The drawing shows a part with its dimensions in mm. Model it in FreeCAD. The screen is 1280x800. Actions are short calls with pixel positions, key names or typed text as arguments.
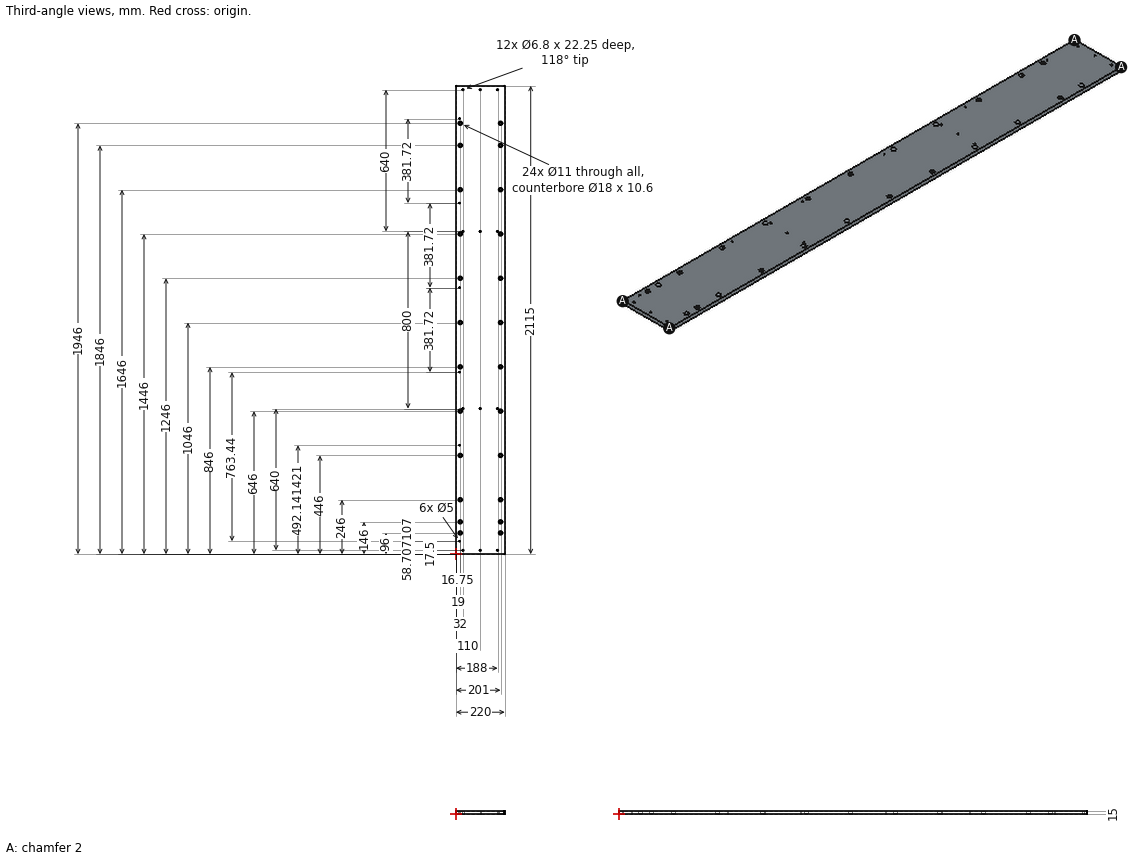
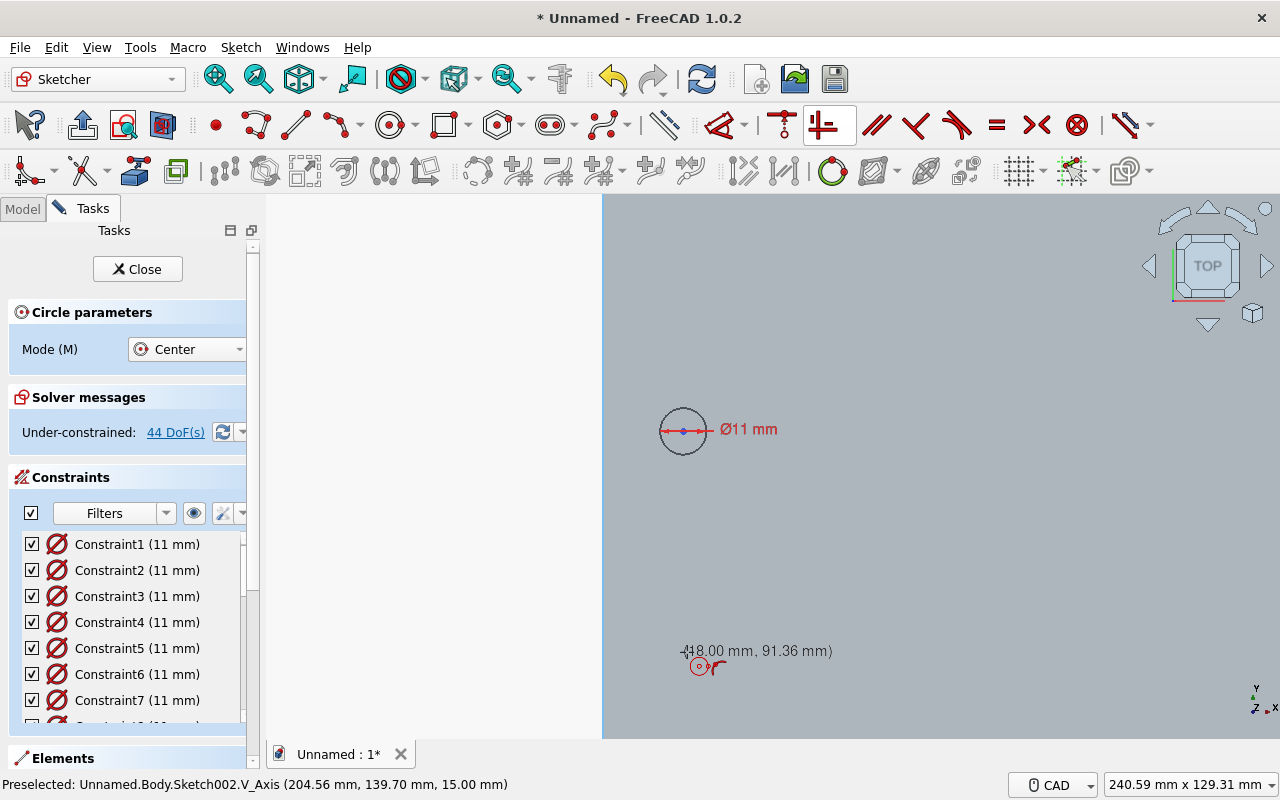
scroll(687, 652, down, 15)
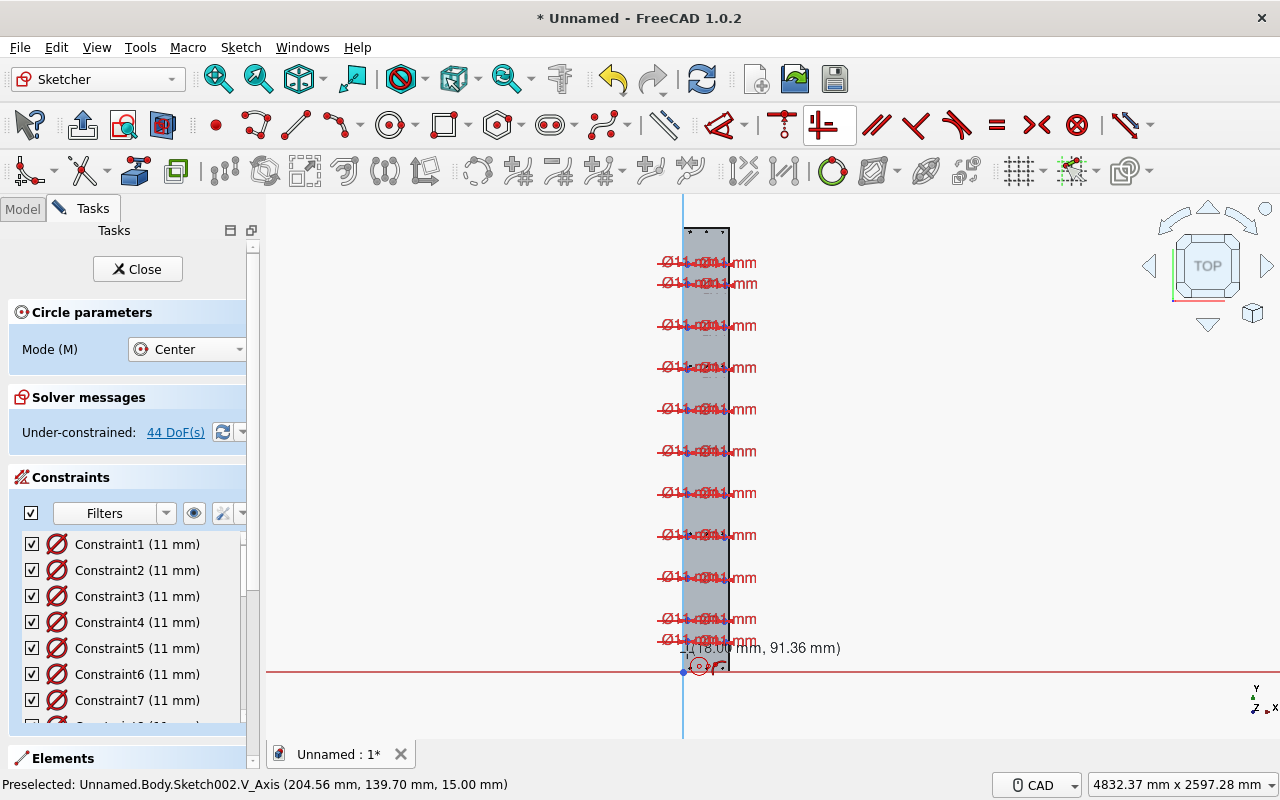
scroll(687, 652, up, 7)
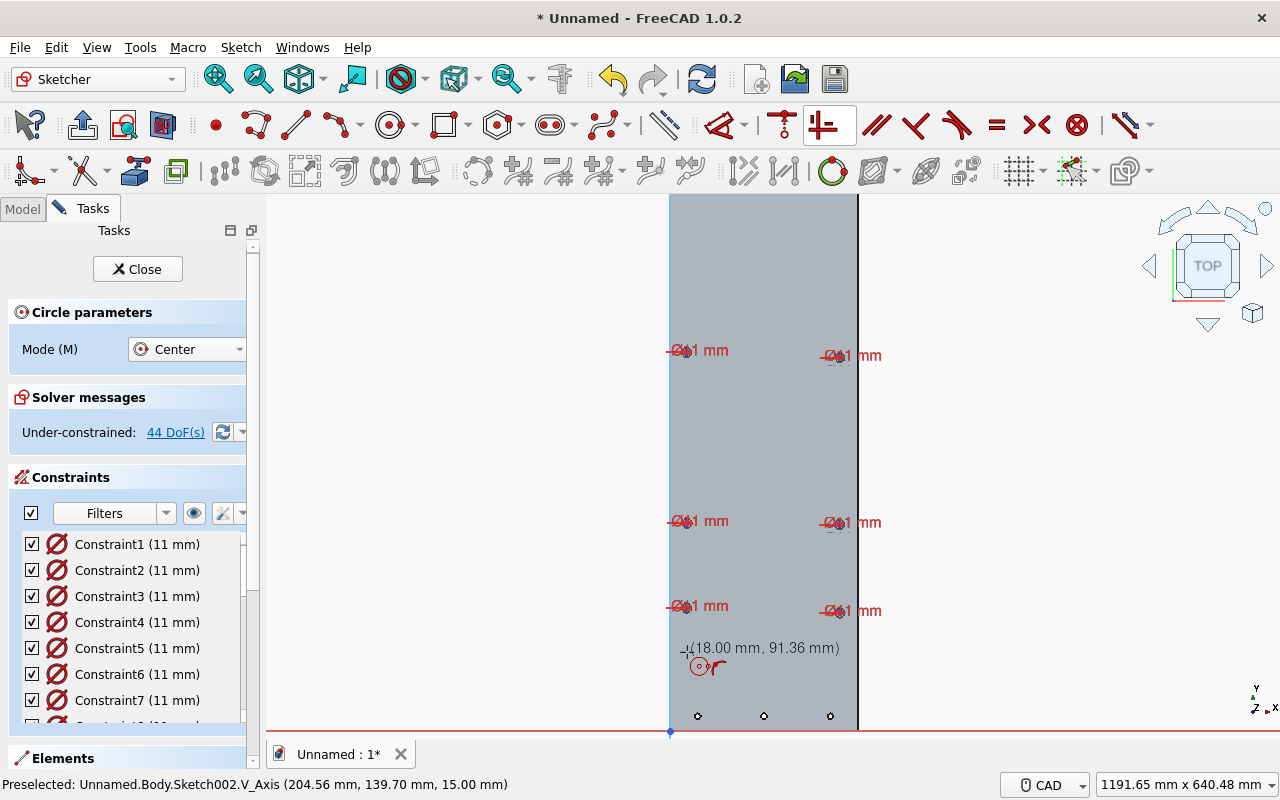
click(687, 650)
move(690, 646)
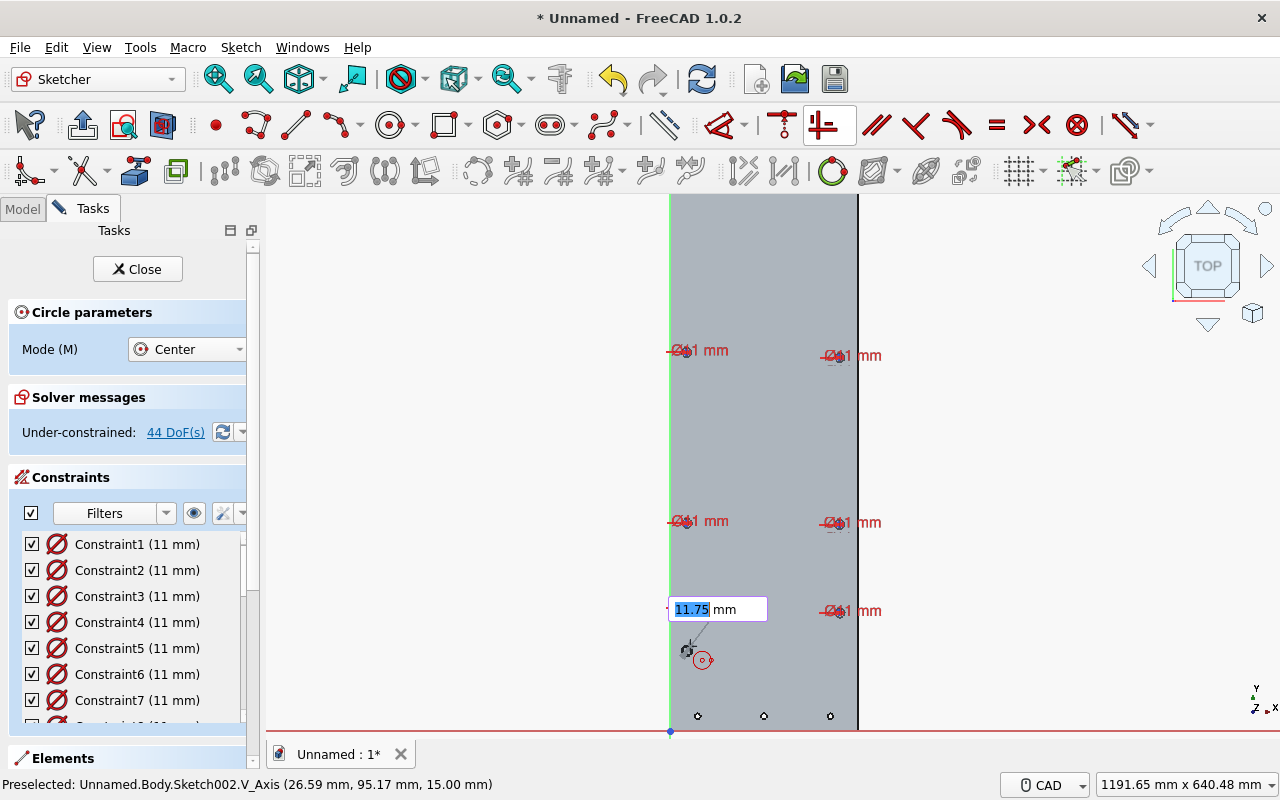
text(11)
key(Return)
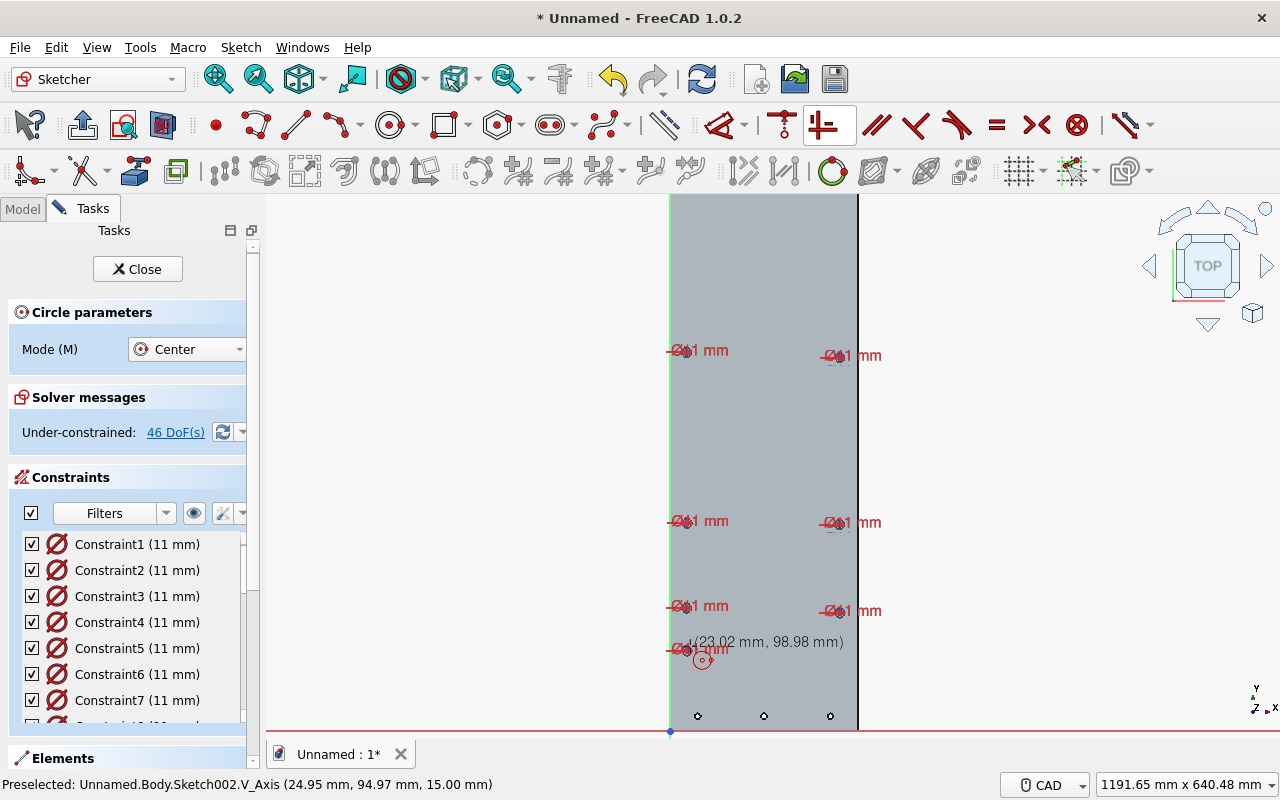
scroll(841, 650, up, 8)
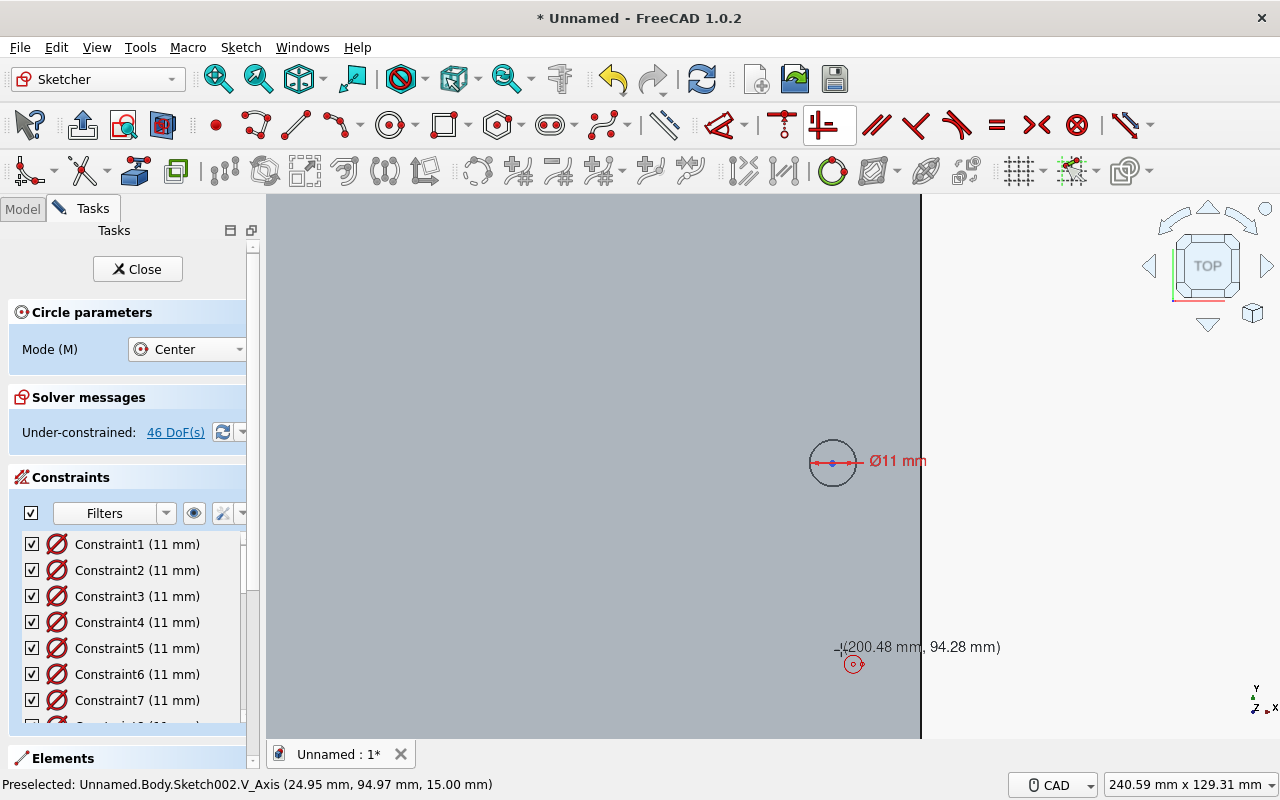
scroll(719, 651, down, 15)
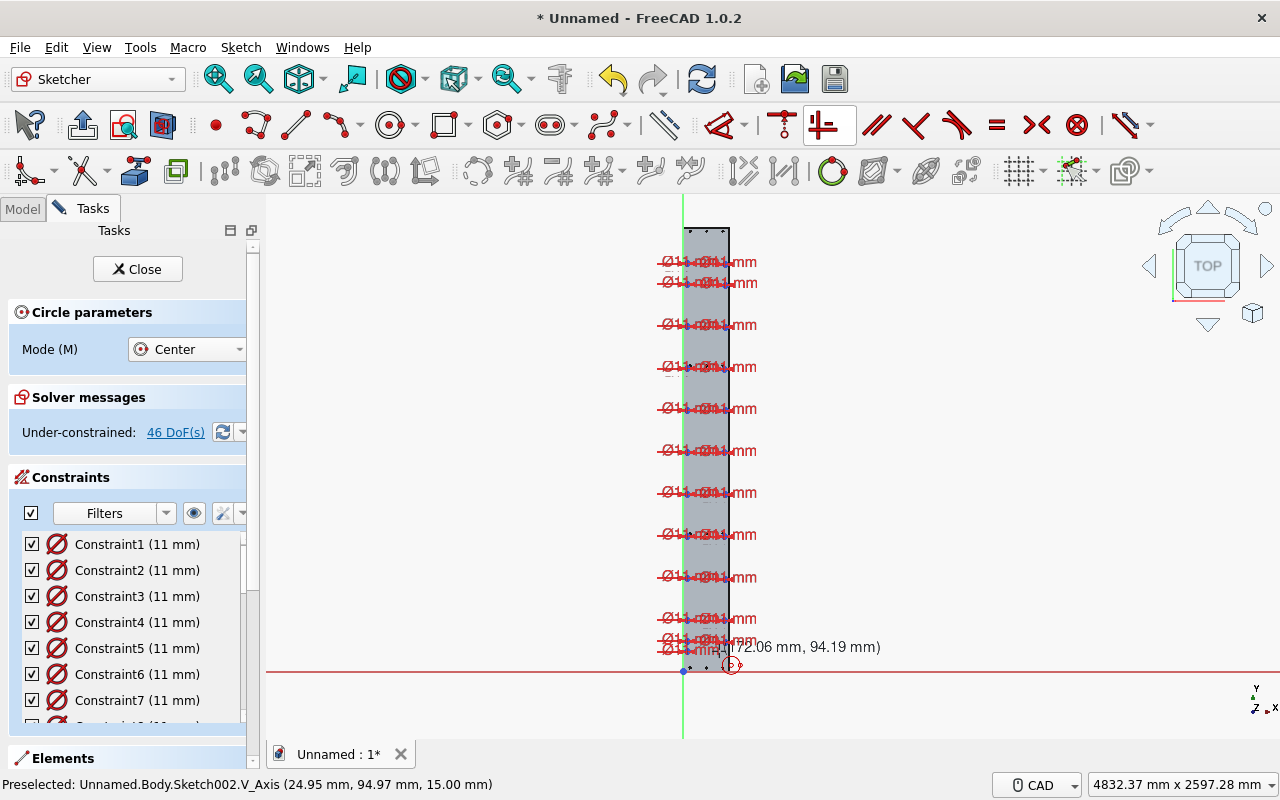
scroll(725, 651, up, 3)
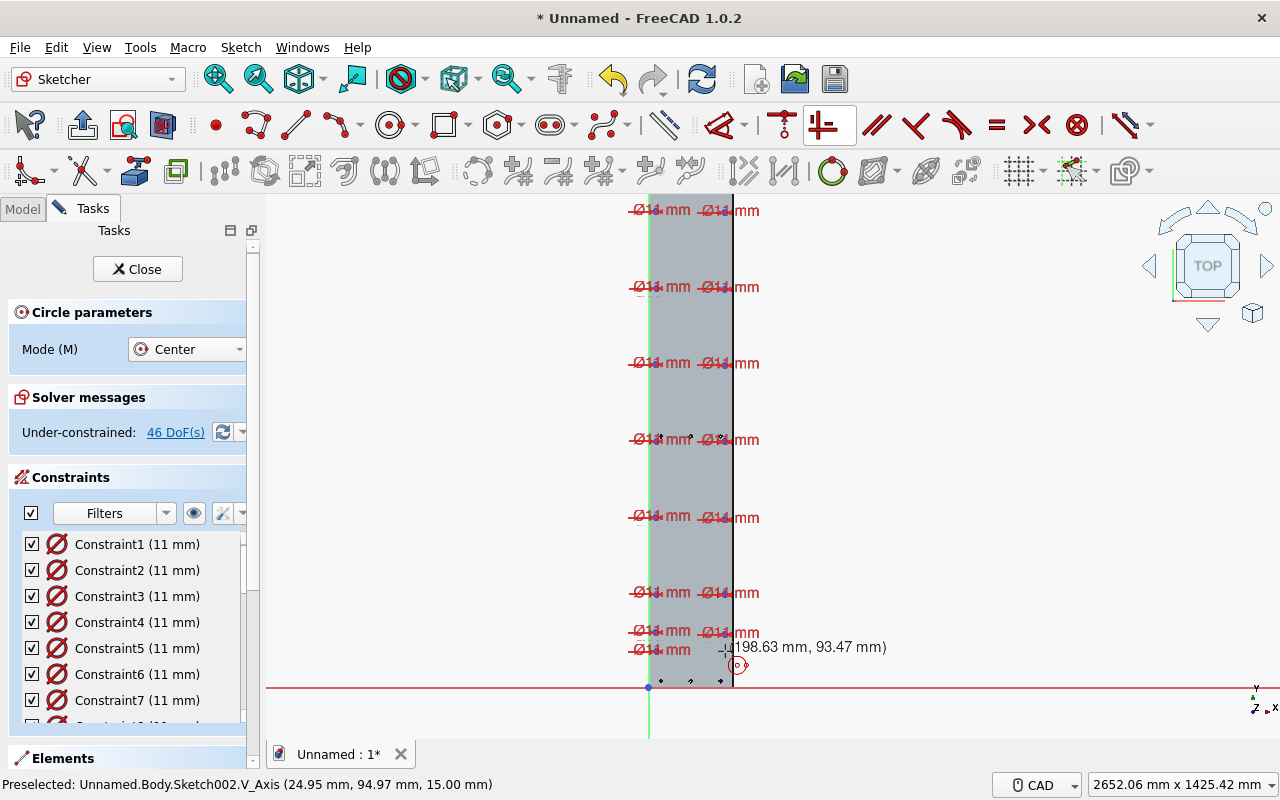
click(726, 651)
move(727, 650)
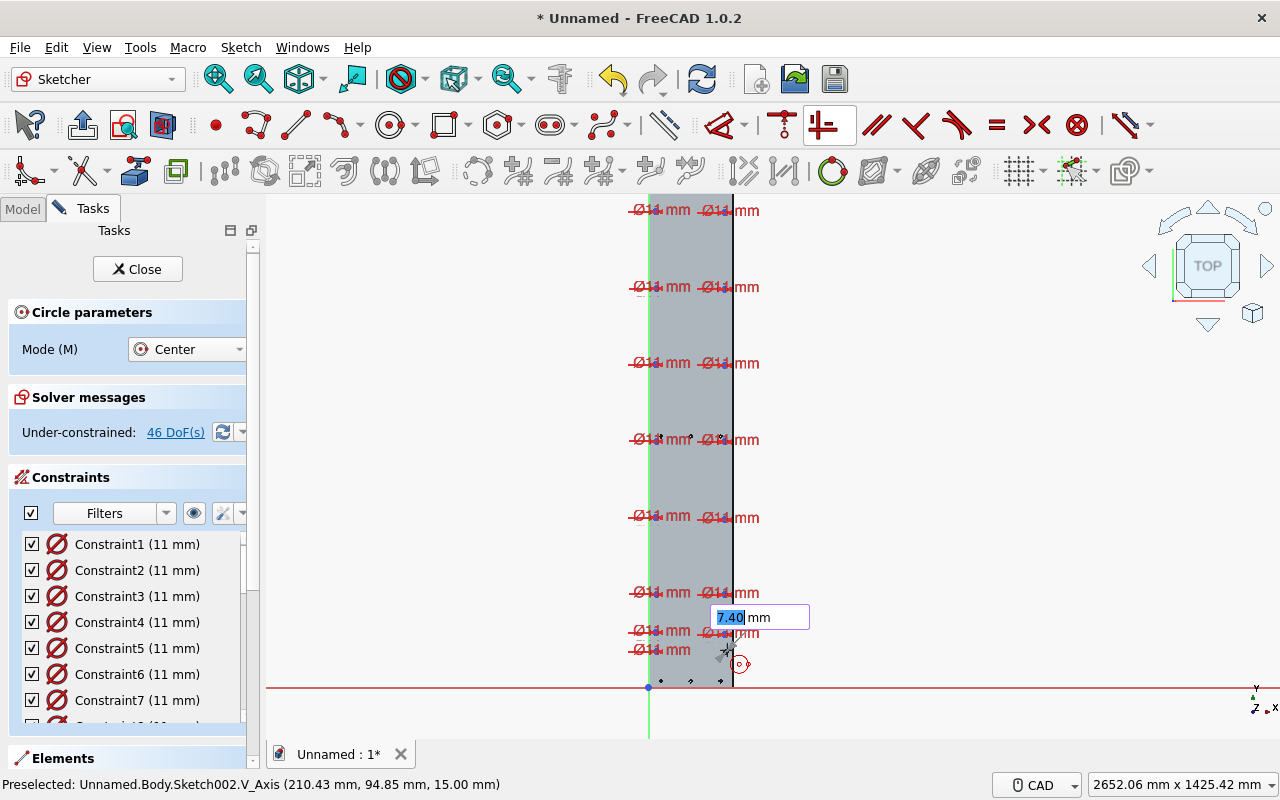
text(11)
key(Return)
key(Escape)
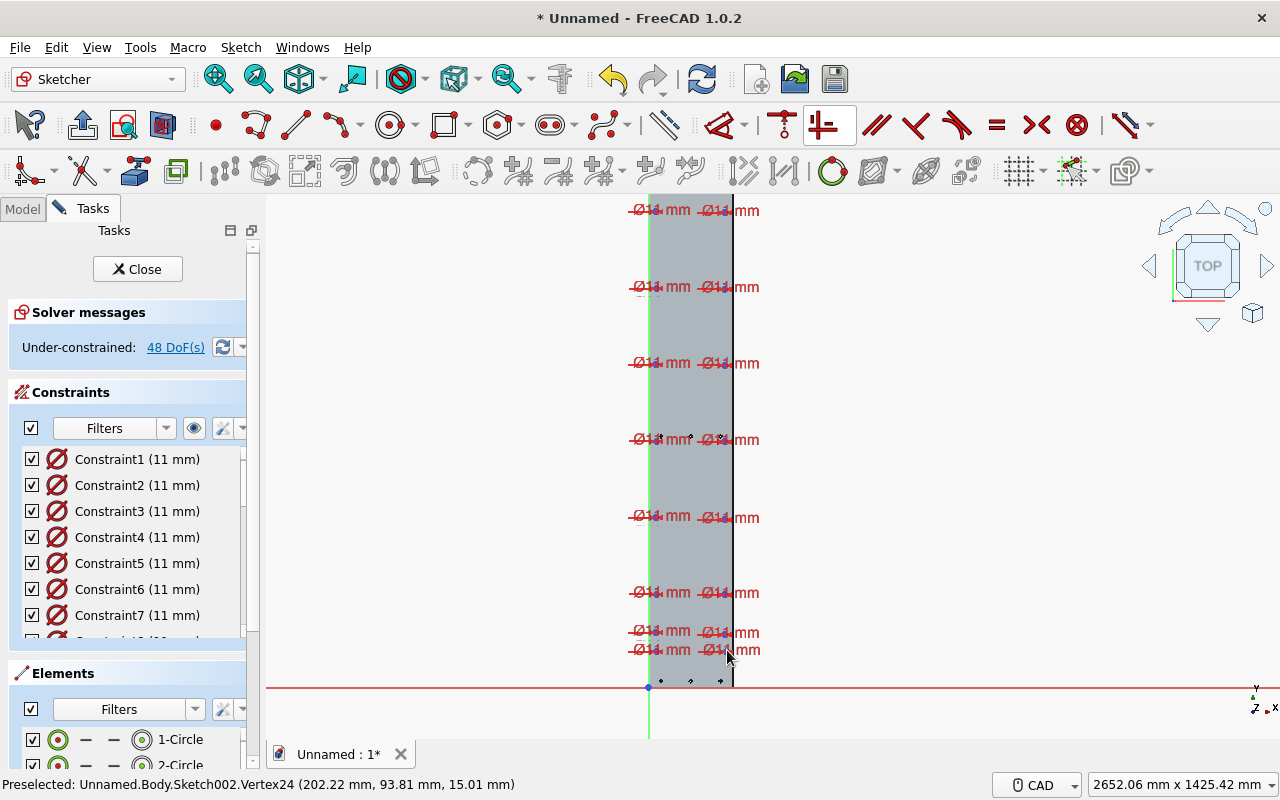
scroll(718, 590, down, 4)